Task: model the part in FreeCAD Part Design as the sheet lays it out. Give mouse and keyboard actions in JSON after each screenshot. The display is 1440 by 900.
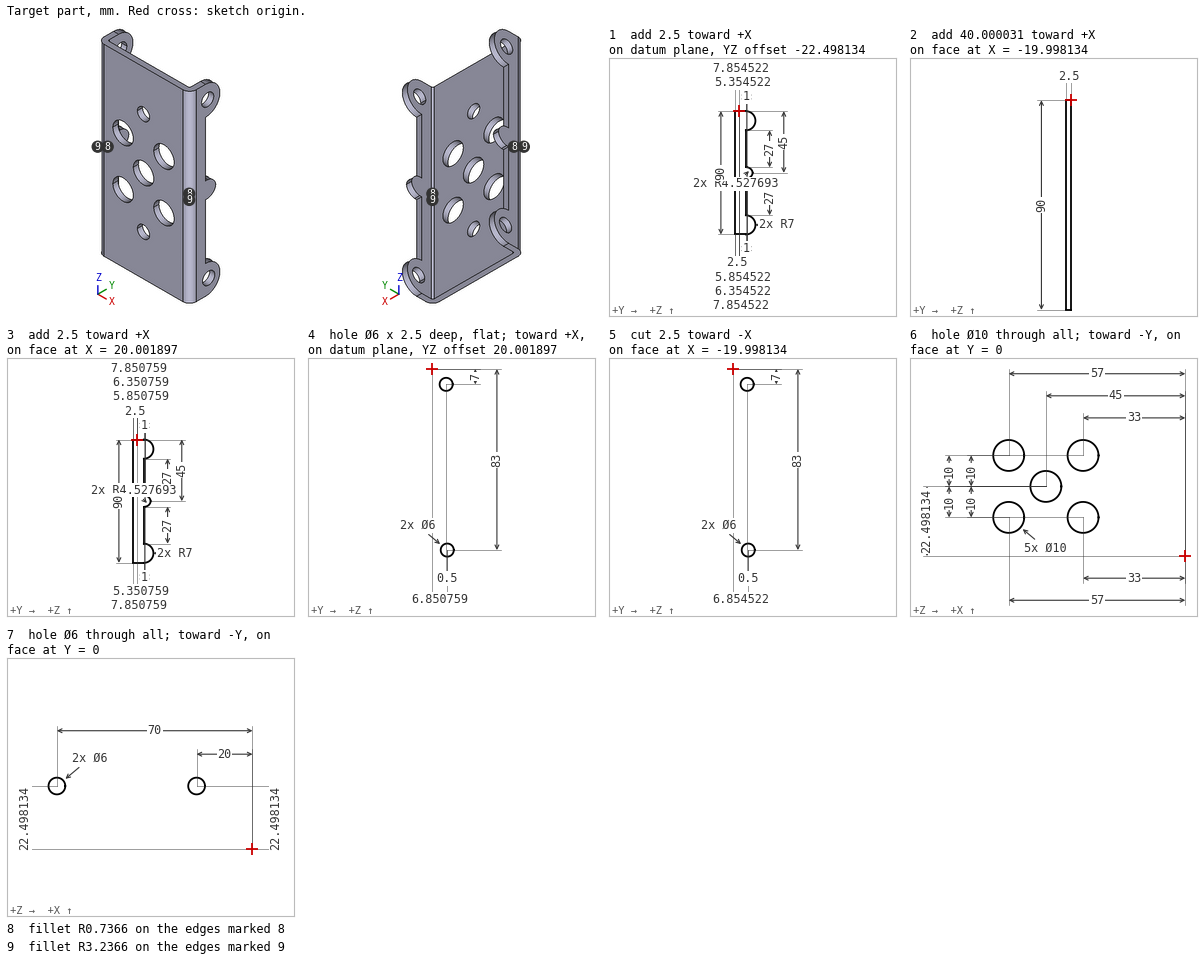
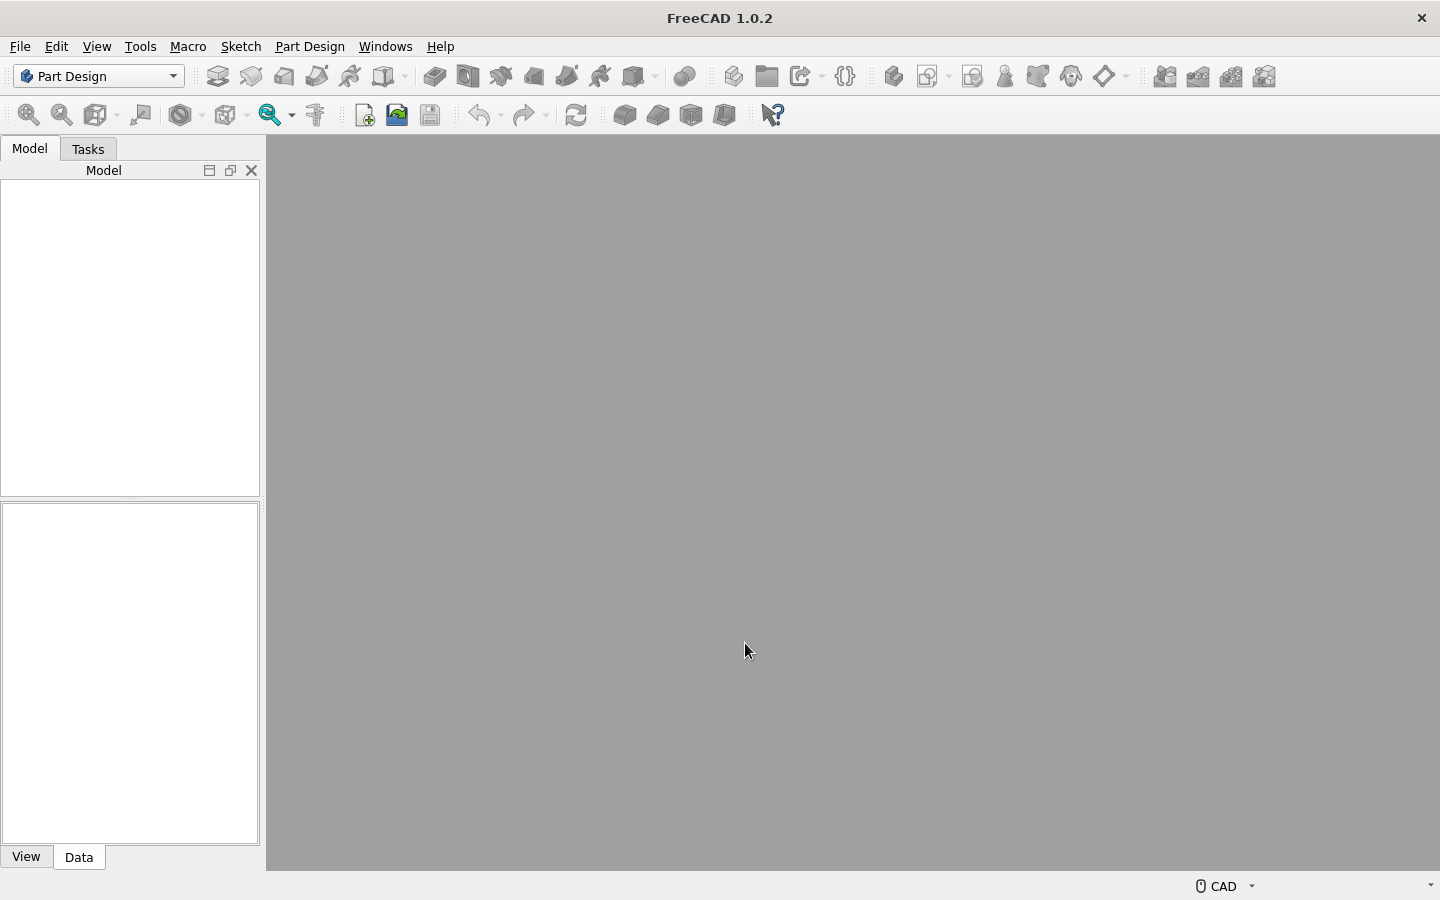
{"action": "left_click", "coordinate": [364, 116]}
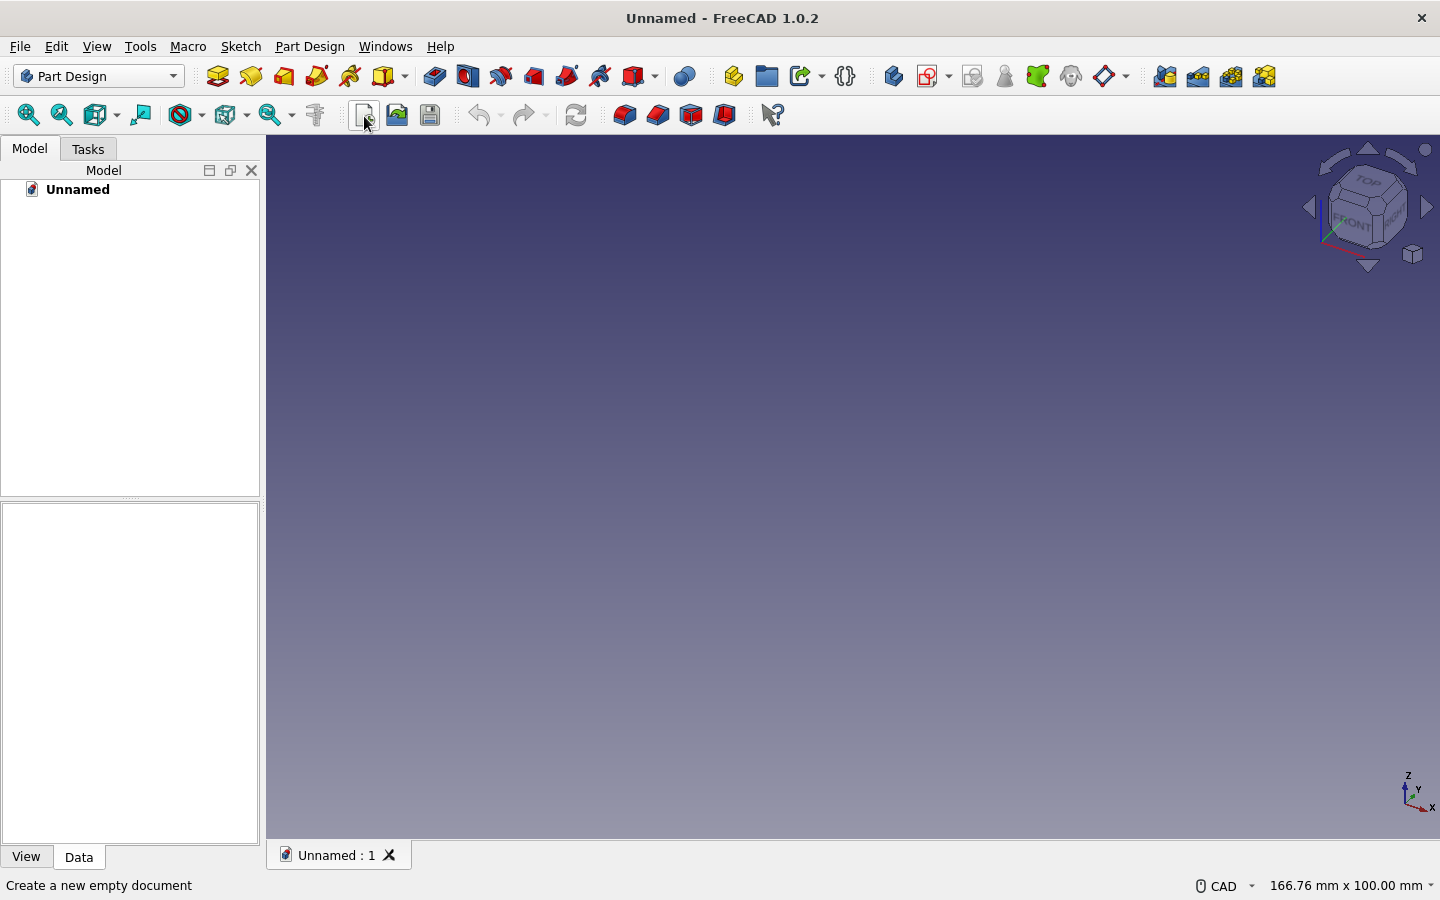
{"action": "left_click", "coordinate": [894, 76]}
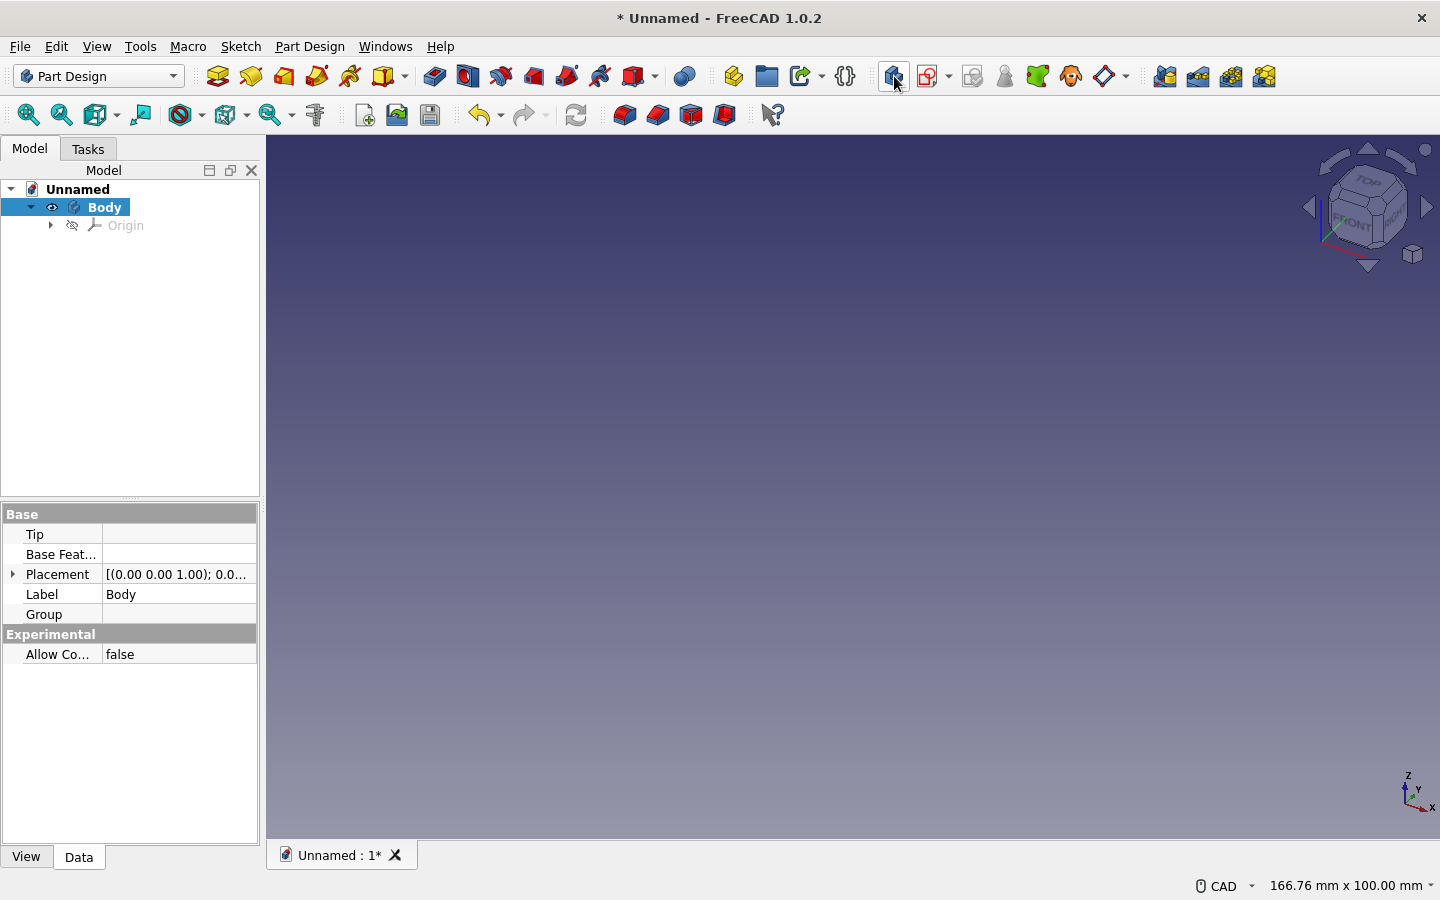
{"action": "left_click", "coordinate": [51, 225]}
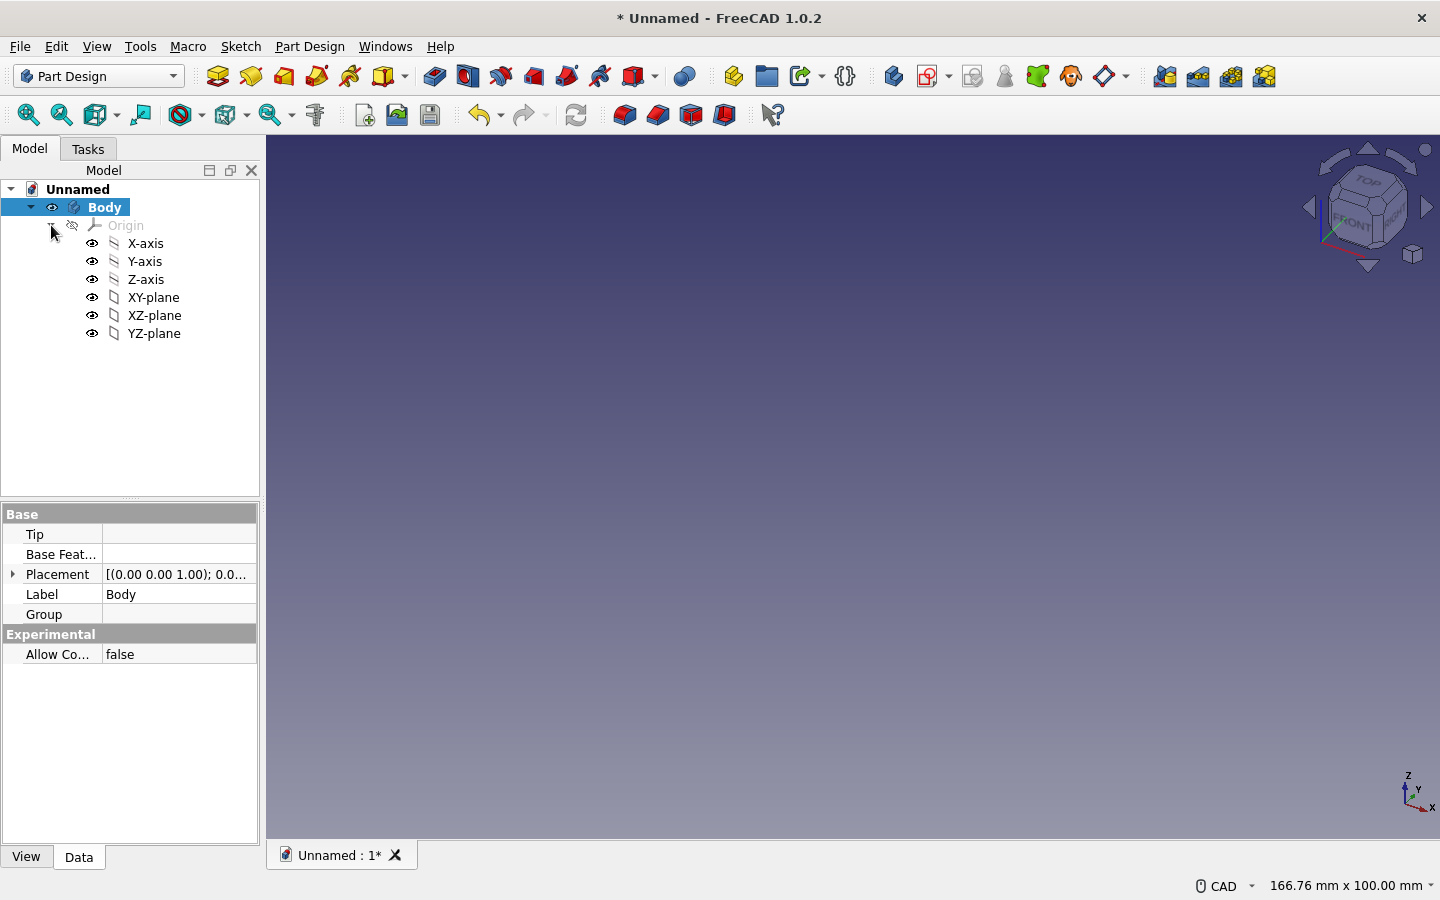
{"action": "left_click", "coordinate": [137, 333]}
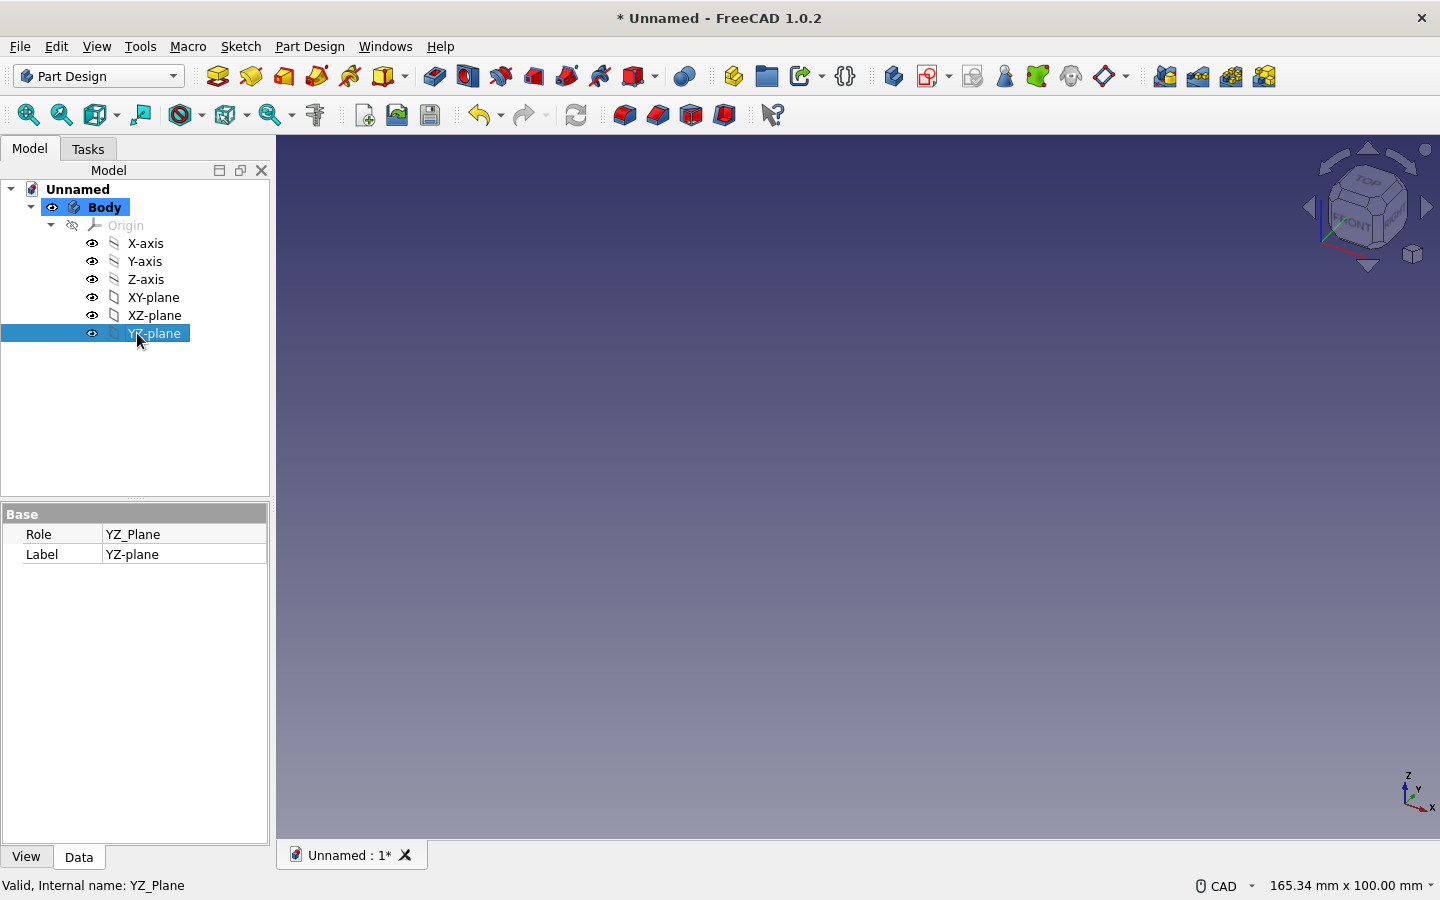
{"action": "left_click", "coordinate": [1104, 76]}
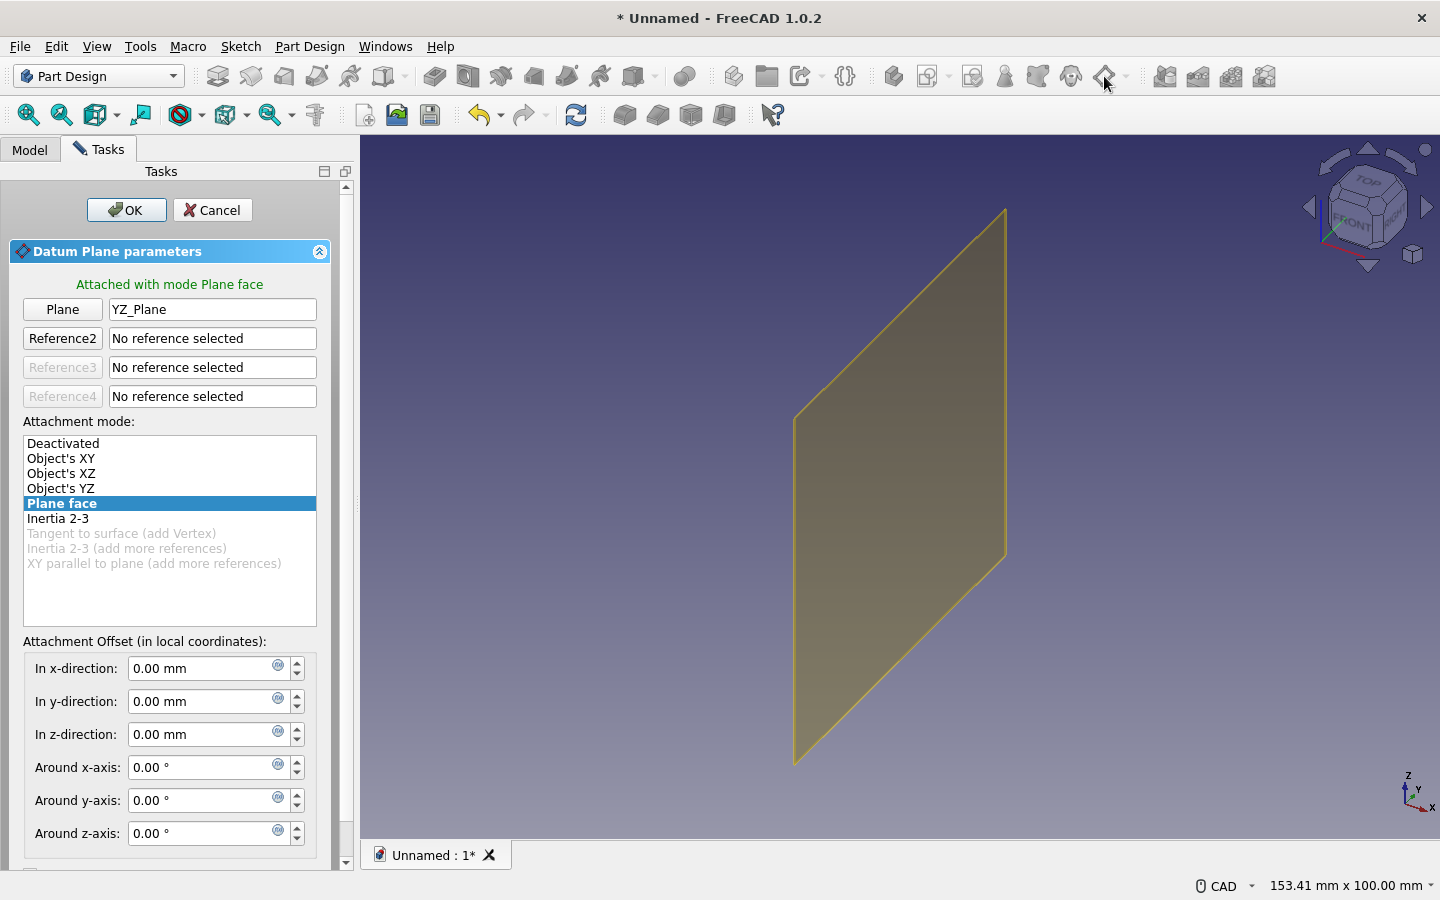
{"action": "triple_click", "coordinate": [210, 734]}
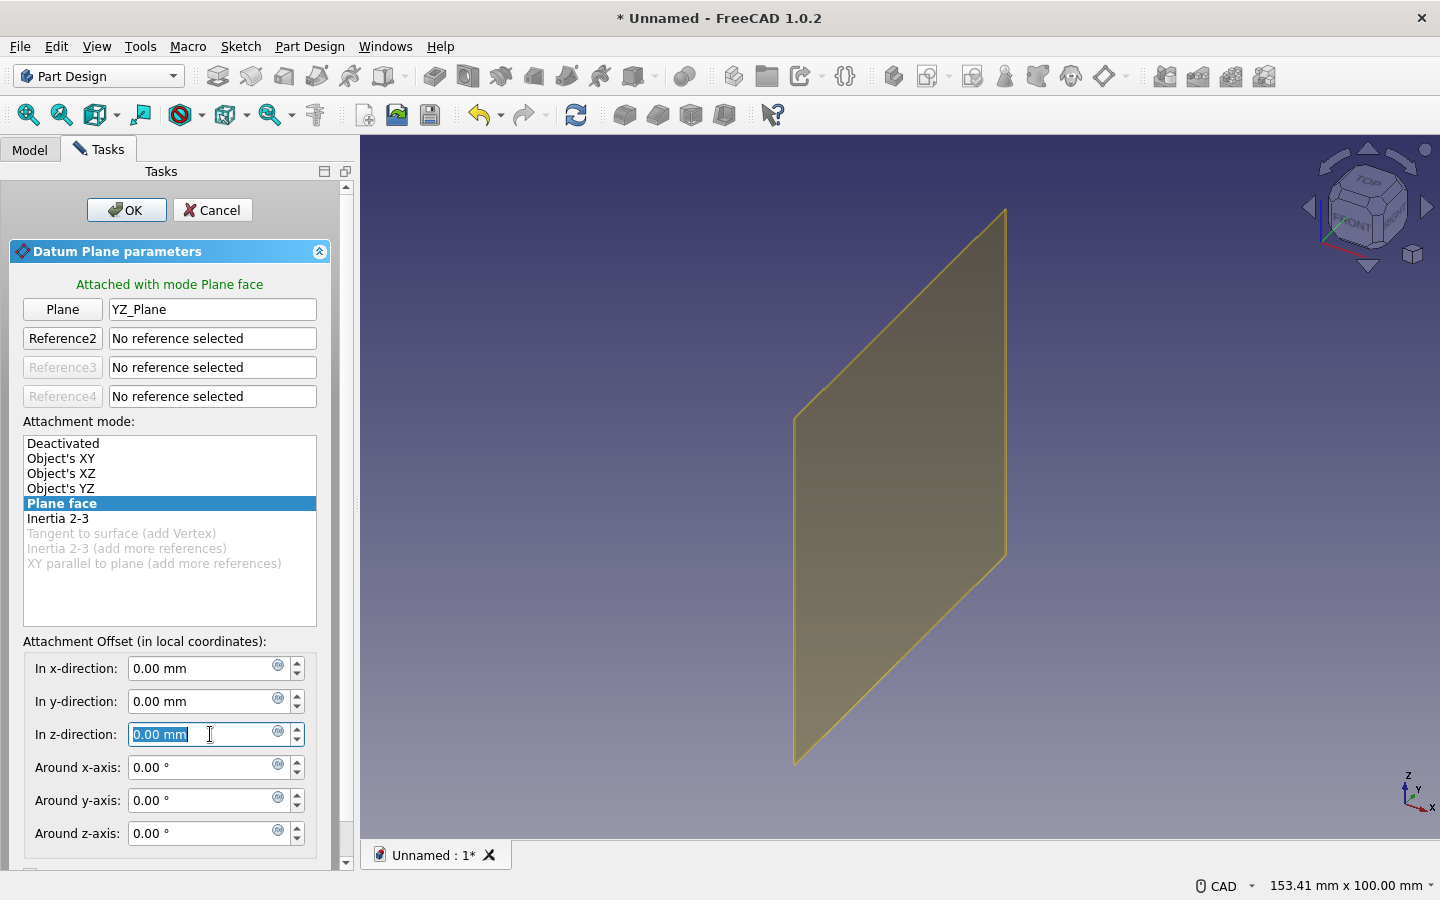
{"action": "type", "text": "-22.498134"}
{"action": "key", "text": "Tab"}